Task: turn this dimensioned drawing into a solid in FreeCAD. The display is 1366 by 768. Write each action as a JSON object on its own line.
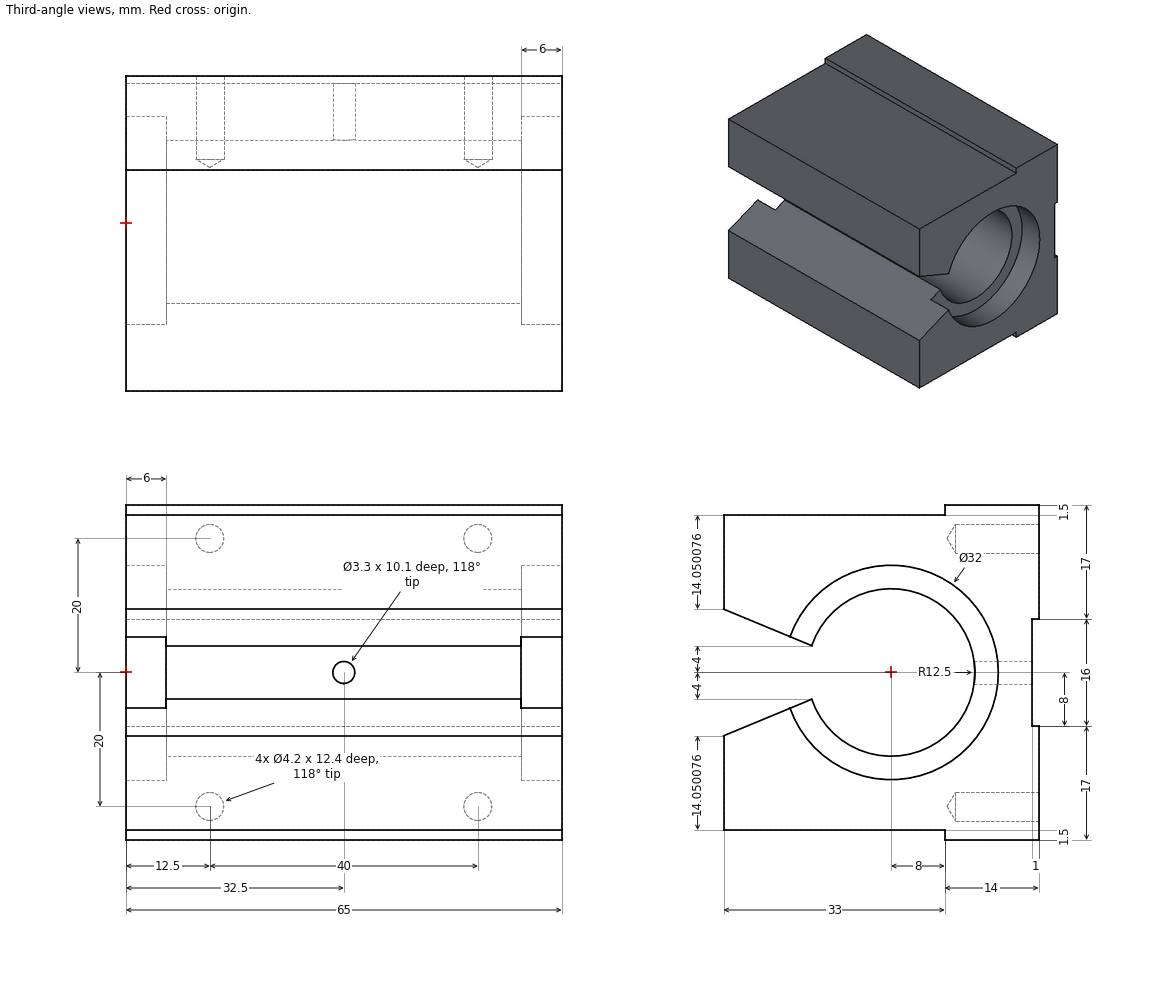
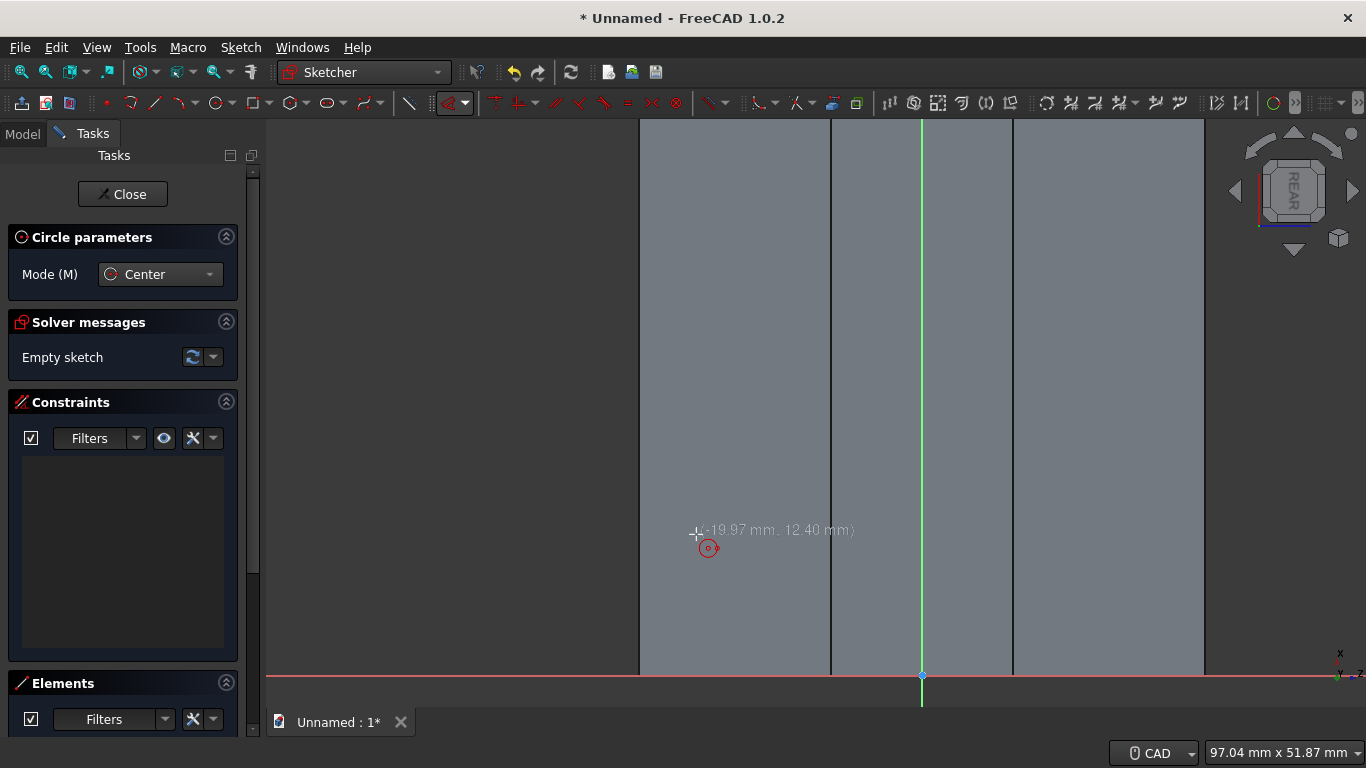
{"action": "left_click", "coordinate": [695, 534]}
{"action": "left_click", "coordinate": [712, 517]}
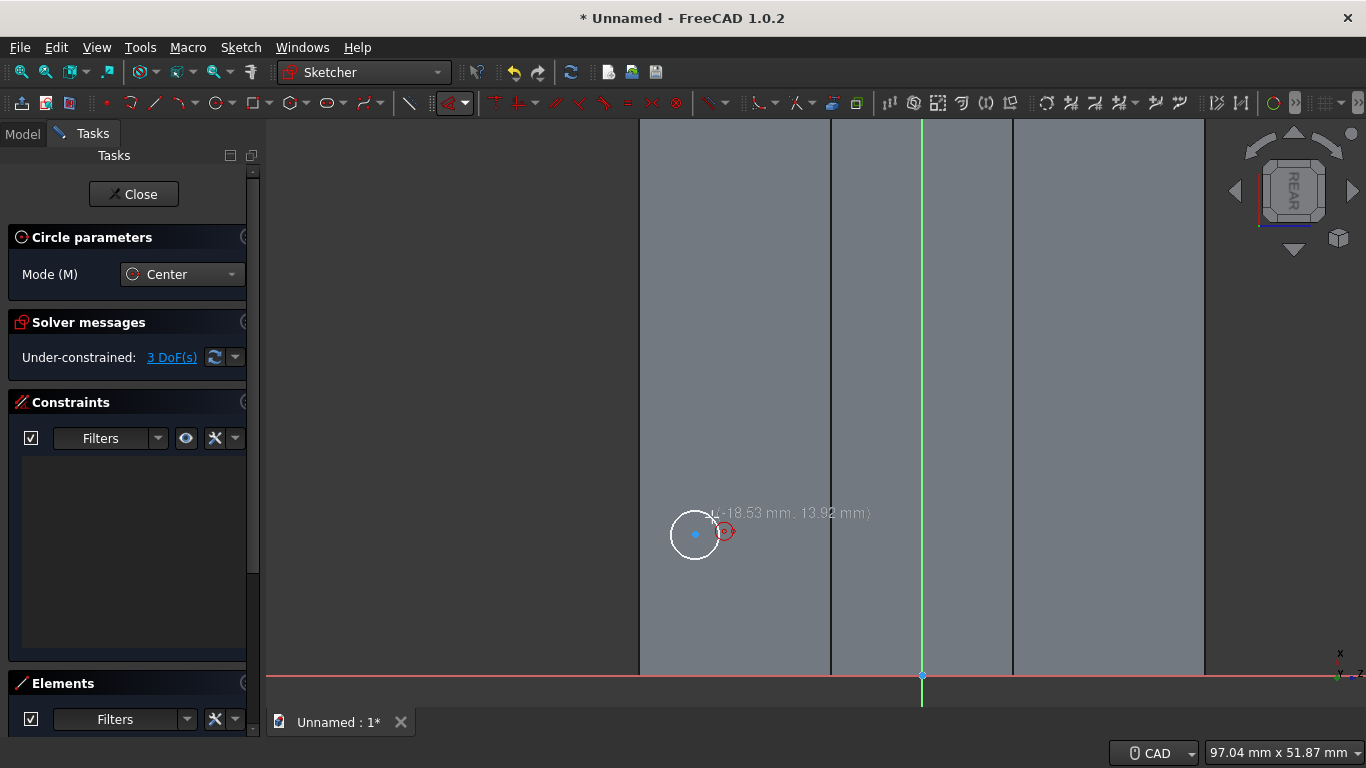
{"action": "scroll", "coordinate": [393, 508], "scroll_direction": "down", "scroll_amount": 2}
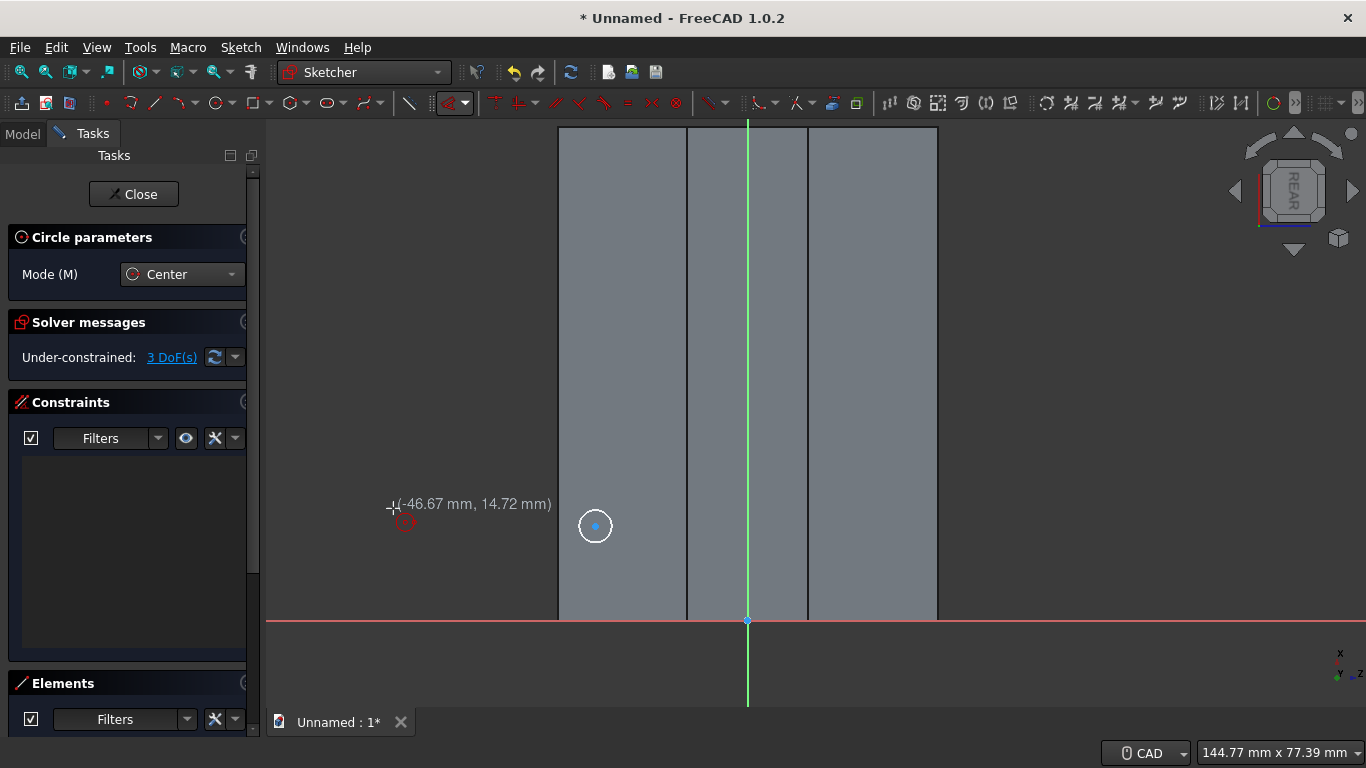
{"action": "scroll", "coordinate": [596, 222], "scroll_direction": "up", "scroll_amount": 2}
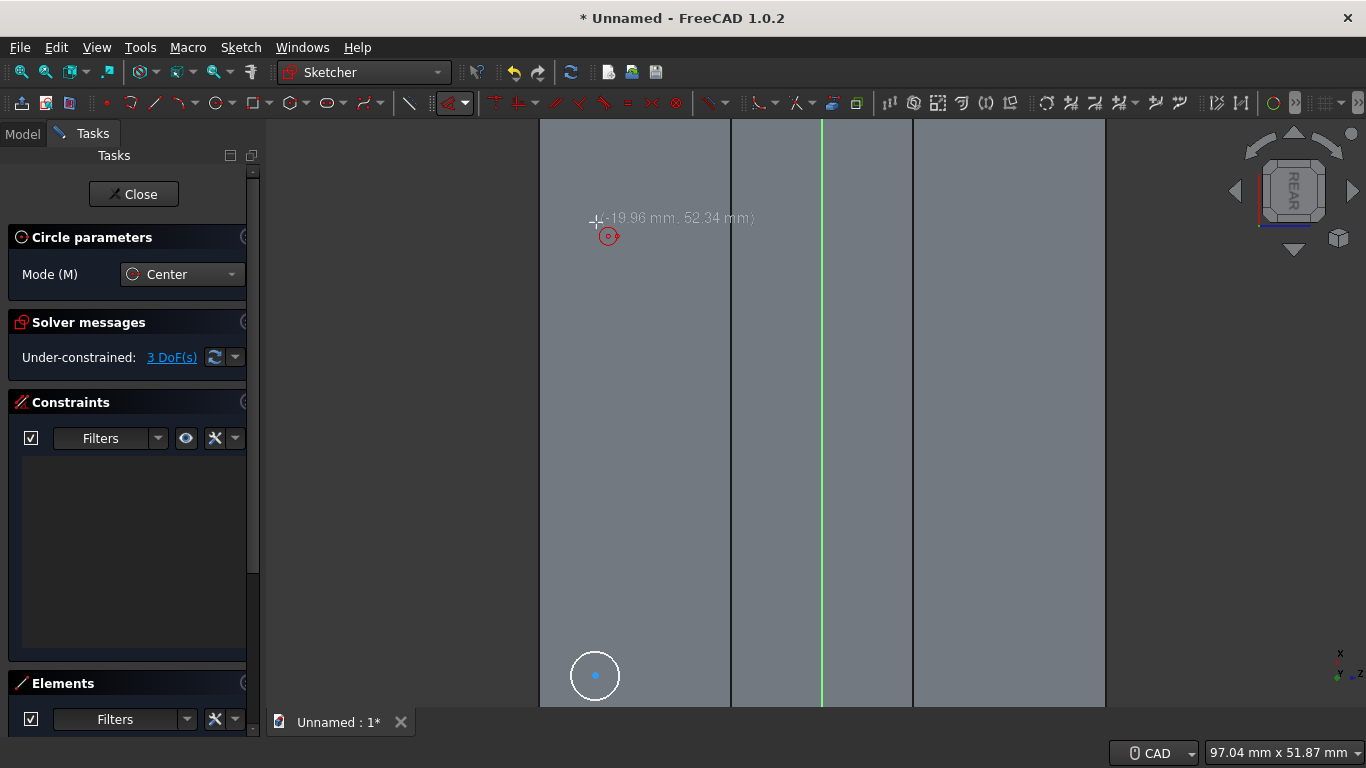
{"action": "left_click", "coordinate": [595, 222]}
{"action": "left_click", "coordinate": [612, 205]}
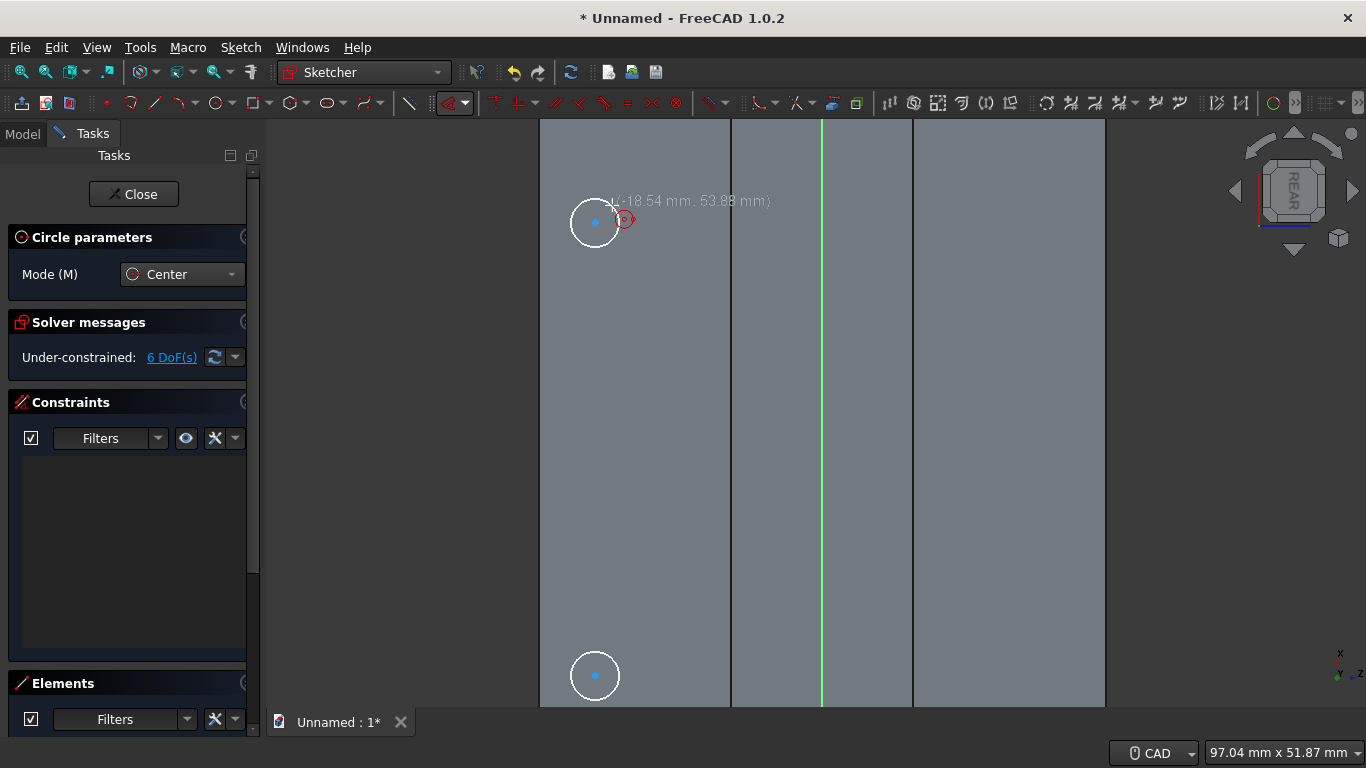
{"action": "left_click", "coordinate": [1049, 675]}
{"action": "left_click", "coordinate": [1066, 658]}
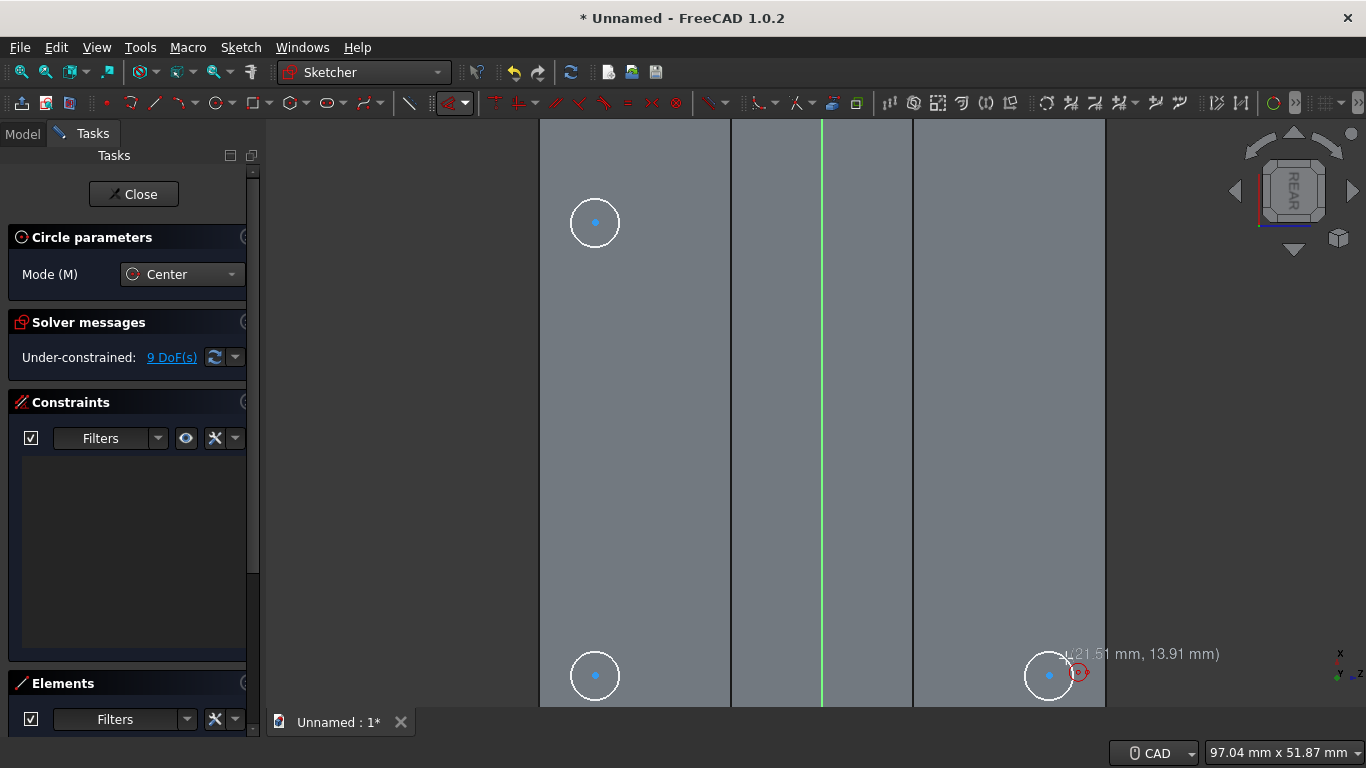
{"action": "left_click", "coordinate": [1049, 222]}
{"action": "left_click", "coordinate": [1066, 205]}
{"action": "key", "text": "Escape"}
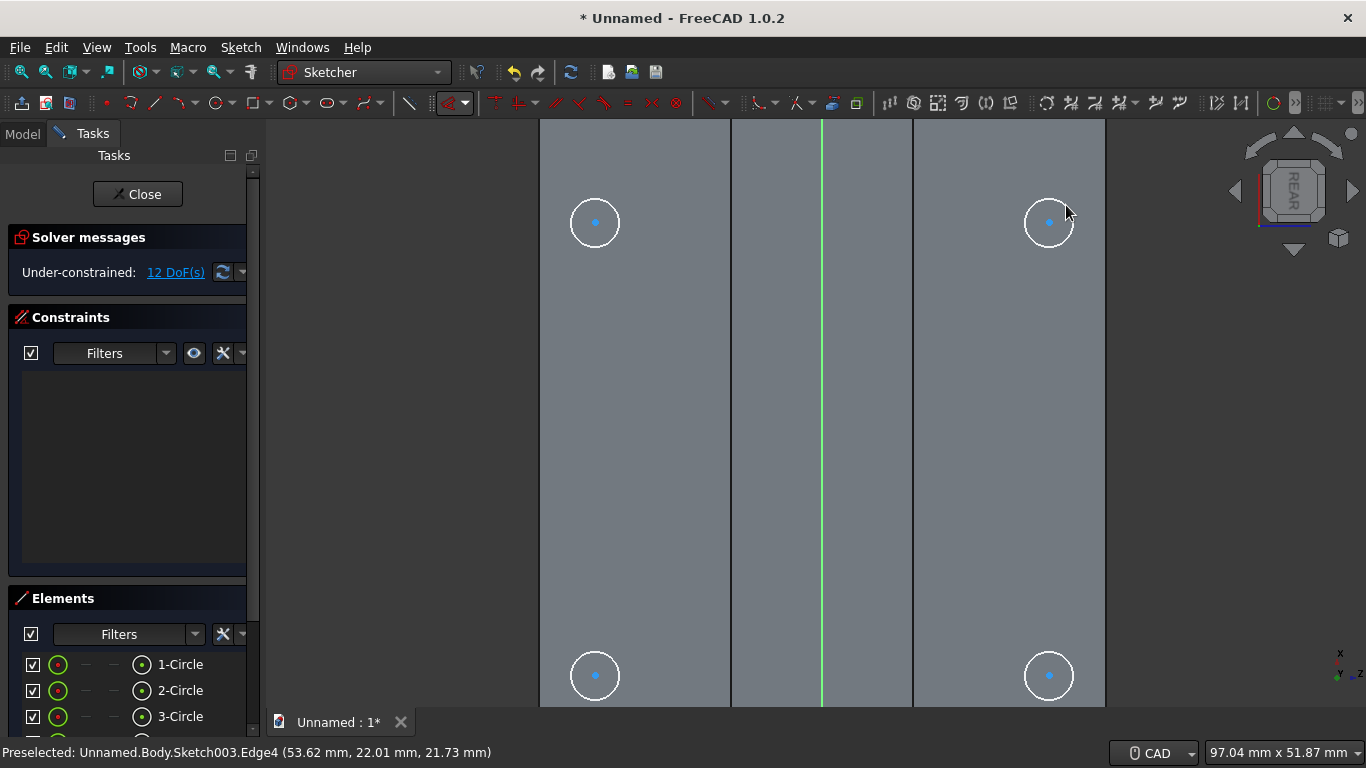
{"action": "left_click", "coordinate": [612, 659]}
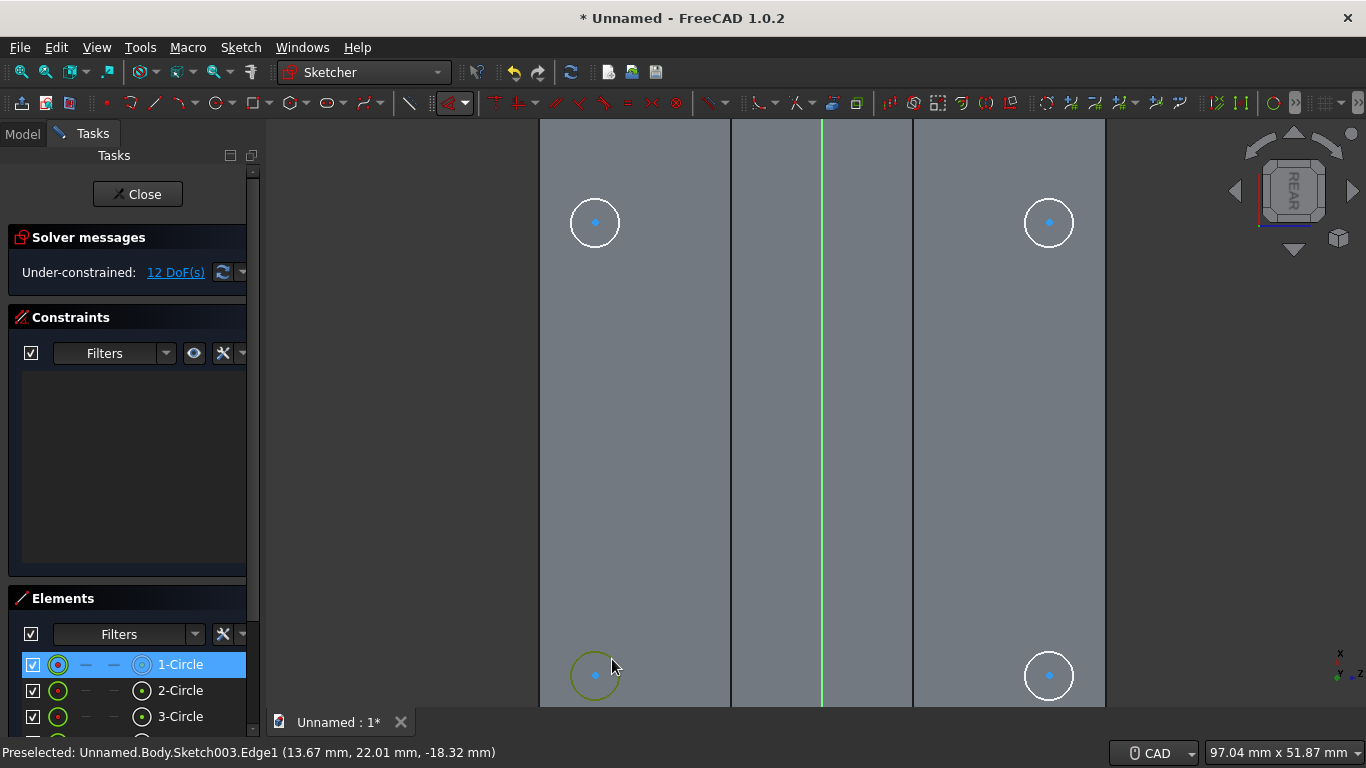
{"action": "left_click", "coordinate": [612, 206]}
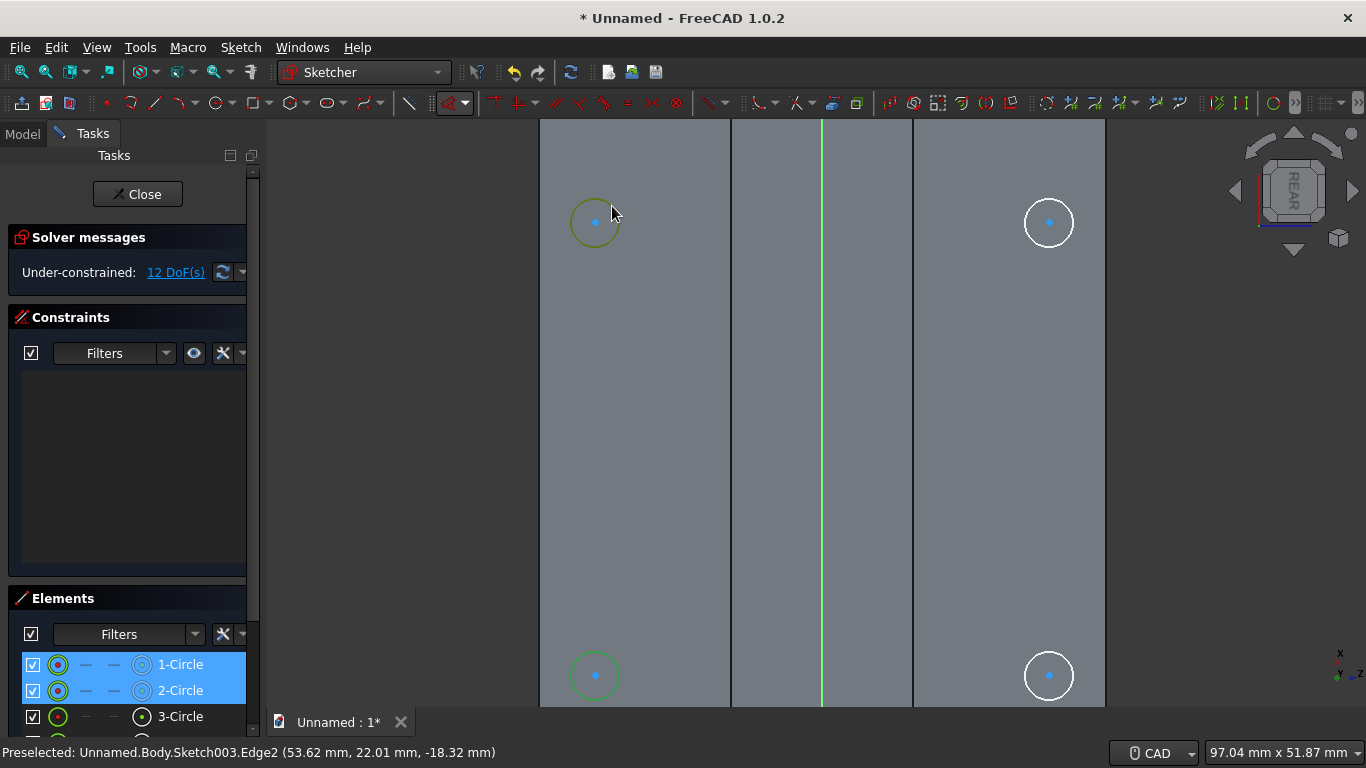
{"action": "left_click", "coordinate": [1066, 659]}